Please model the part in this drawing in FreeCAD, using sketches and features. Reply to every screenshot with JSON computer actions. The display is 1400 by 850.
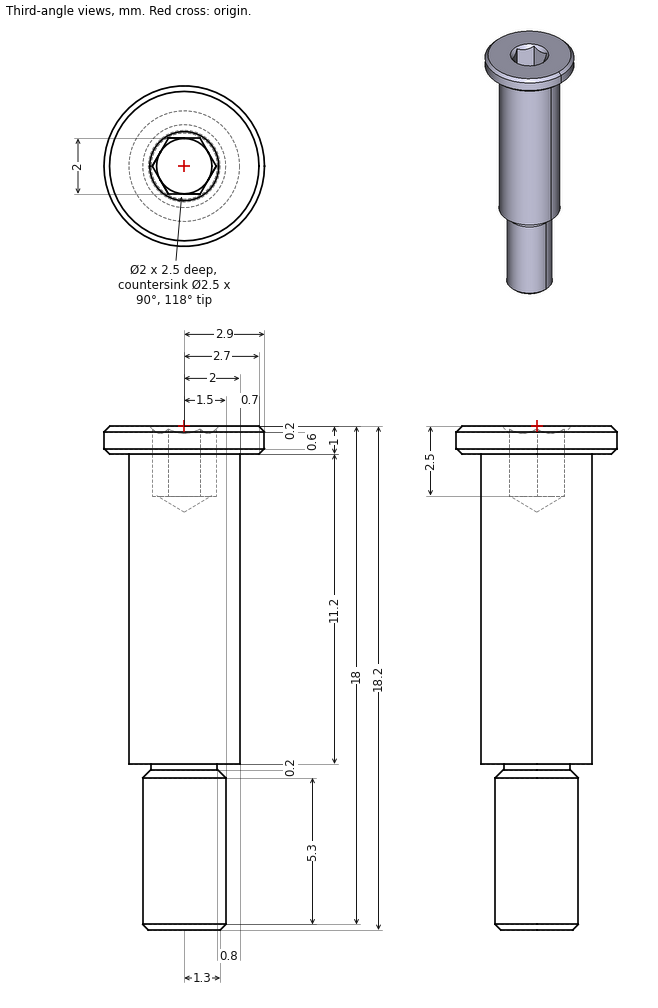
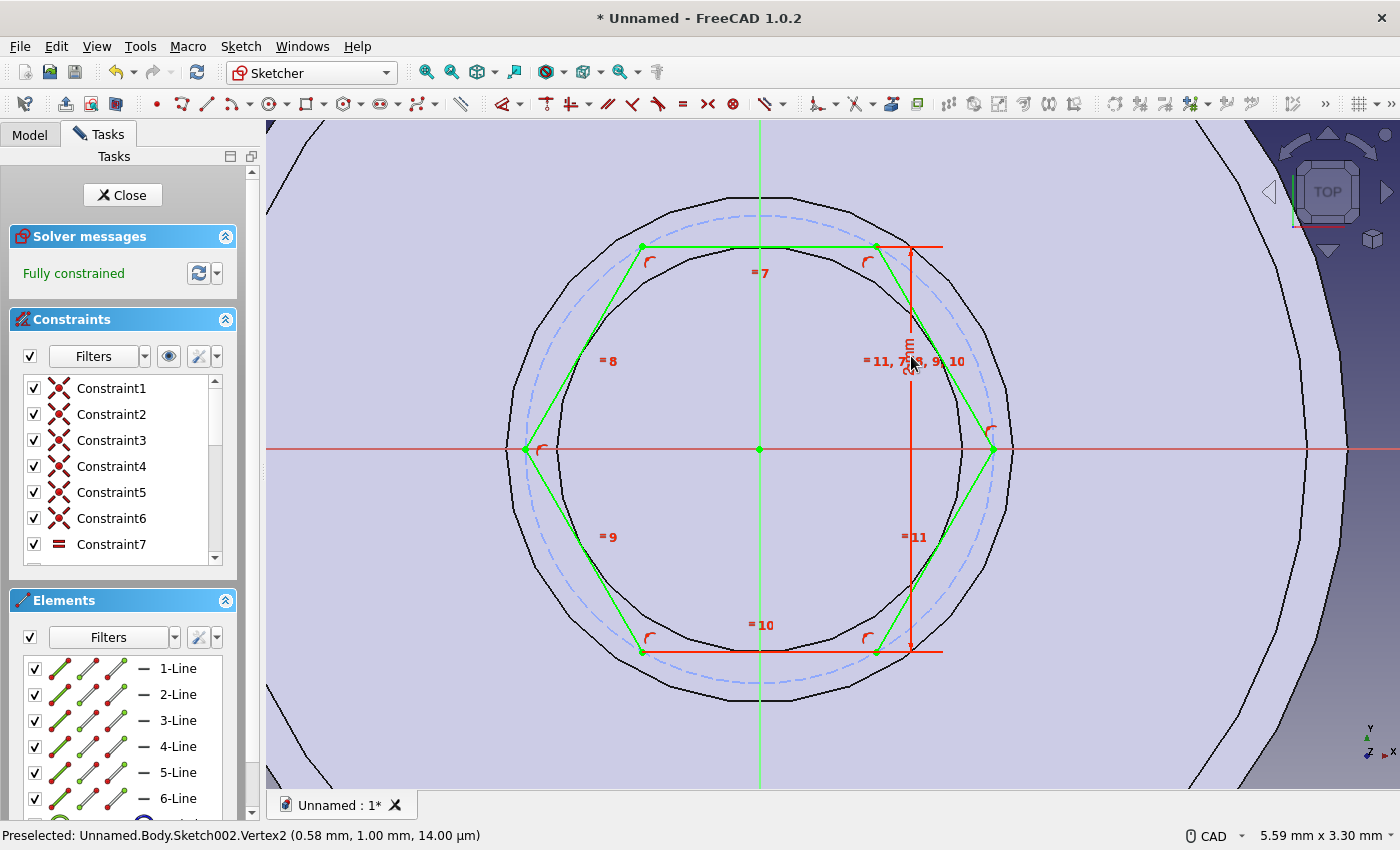
{"action": "left_click", "coordinate": [123, 195]}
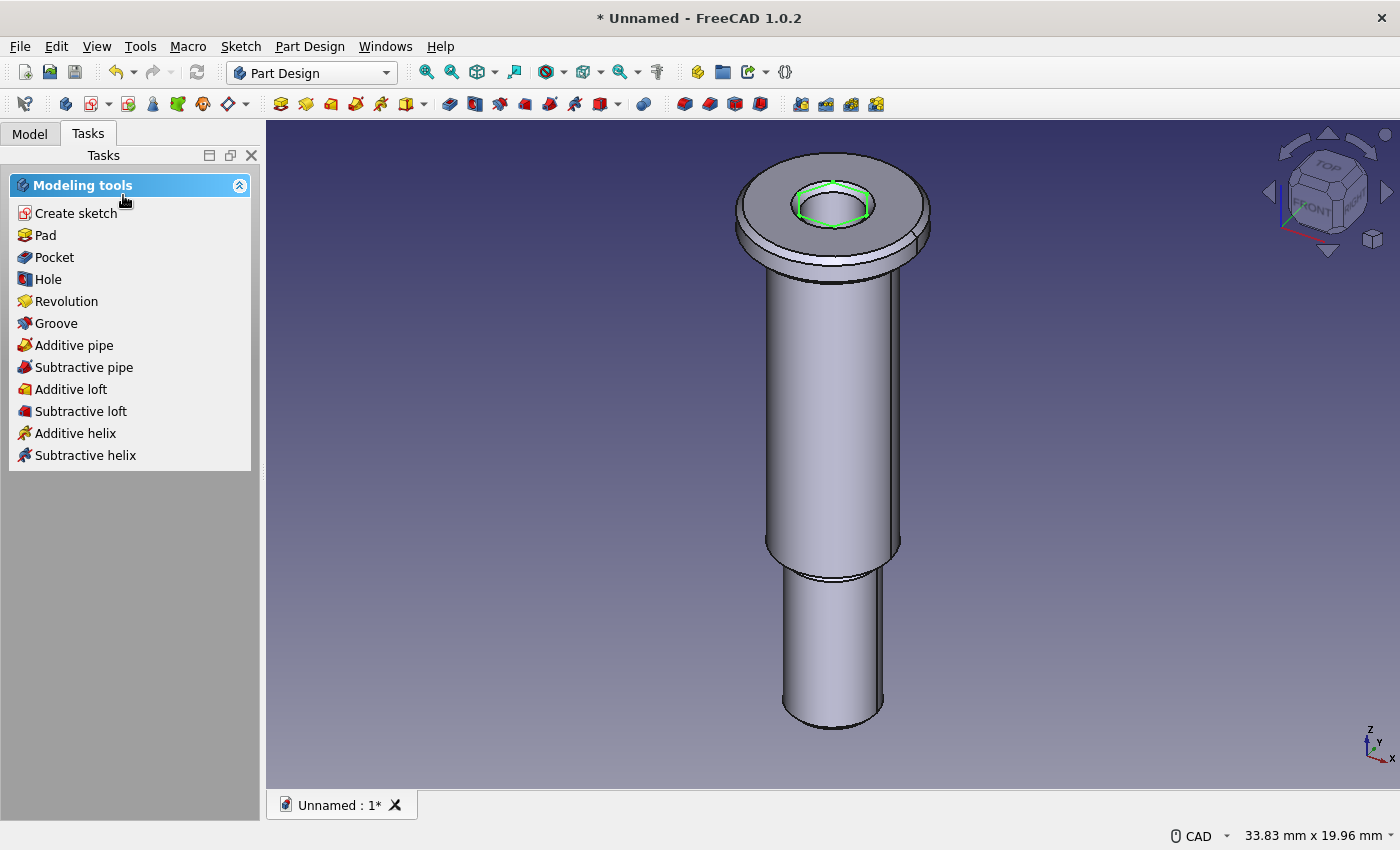
{"action": "left_click", "coordinate": [450, 104]}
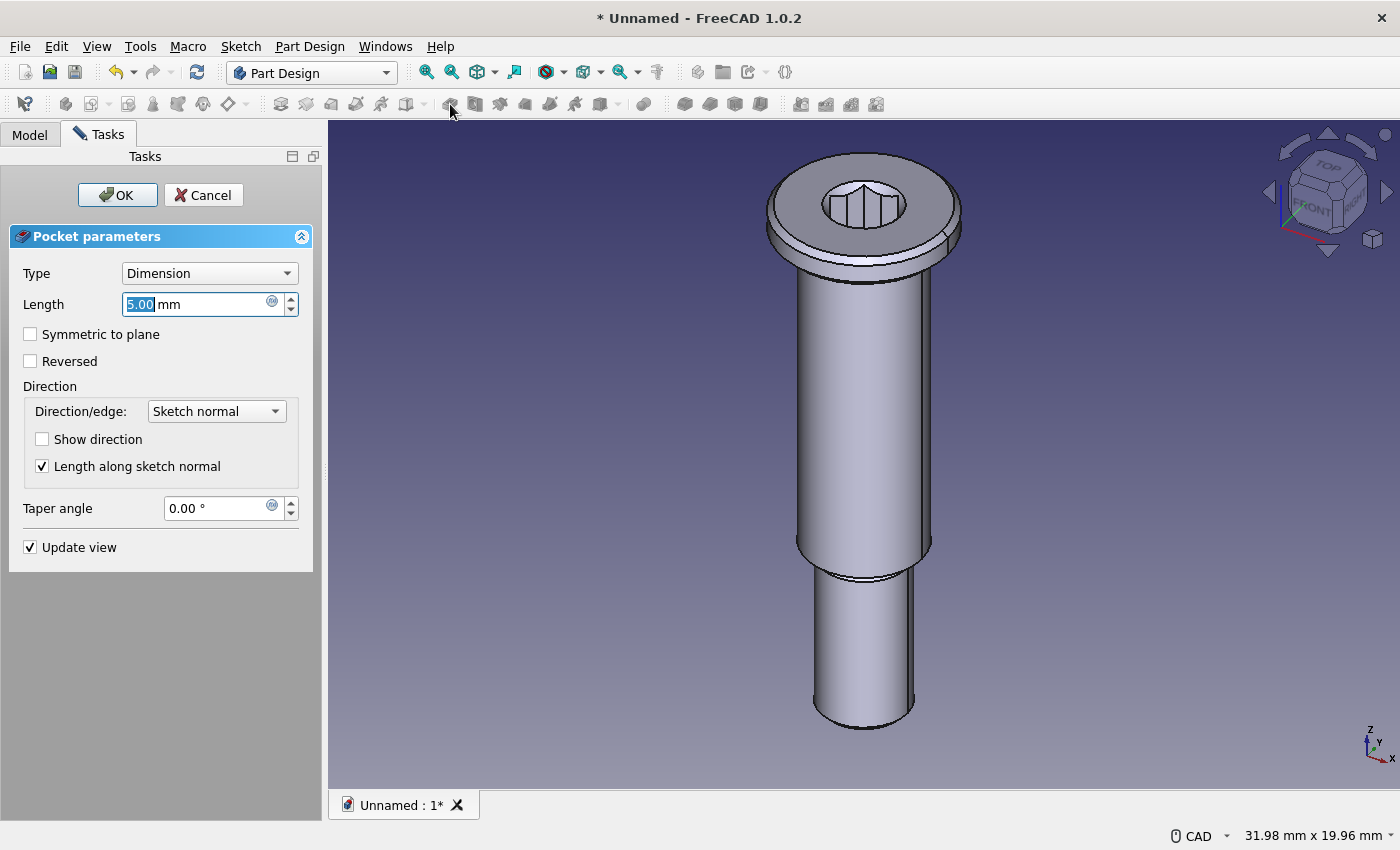
{"action": "type", "text": "2.5"}
{"action": "key", "text": "Tab"}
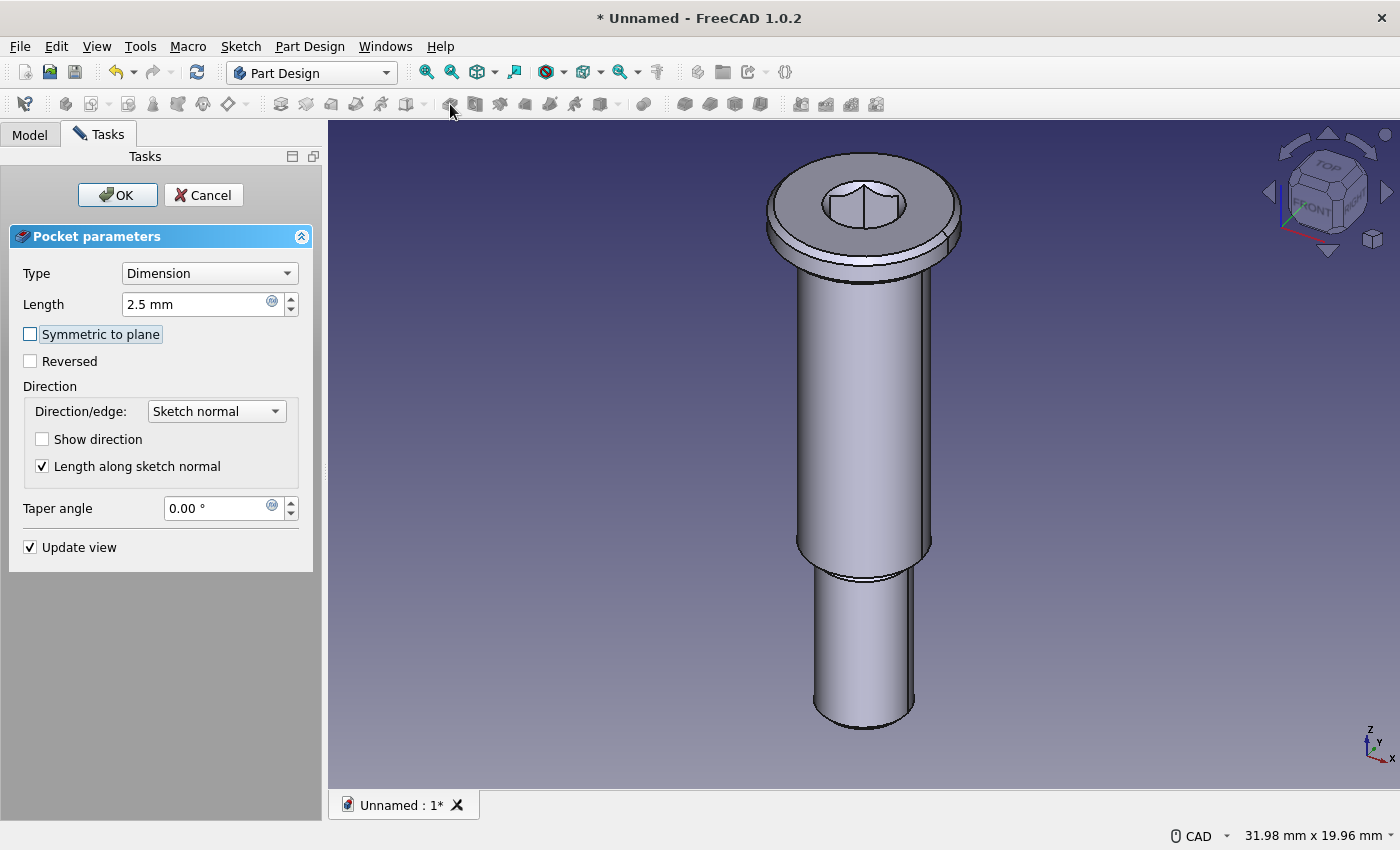
{"action": "left_click", "coordinate": [118, 195]}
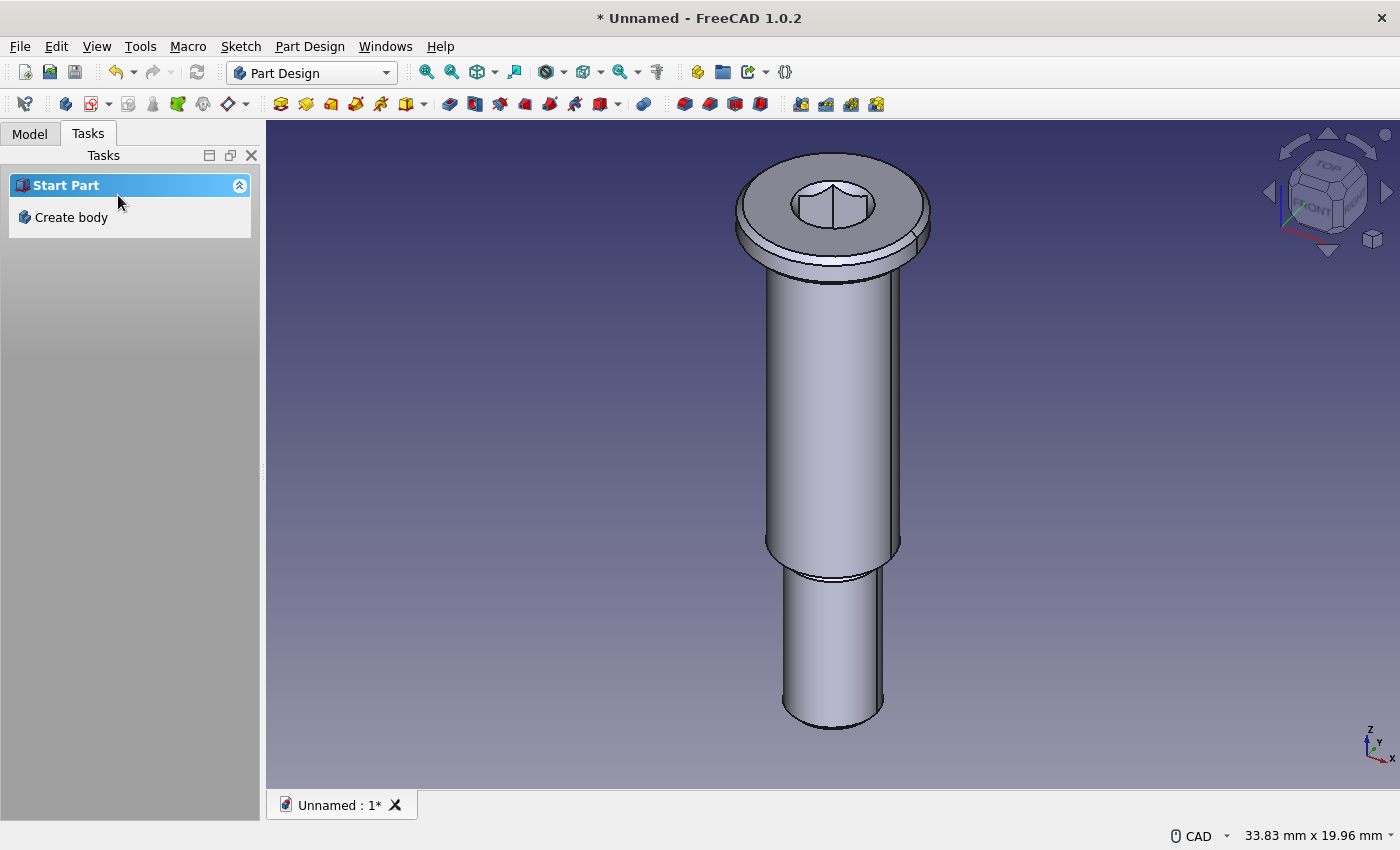
{"action": "key", "text": "0"}